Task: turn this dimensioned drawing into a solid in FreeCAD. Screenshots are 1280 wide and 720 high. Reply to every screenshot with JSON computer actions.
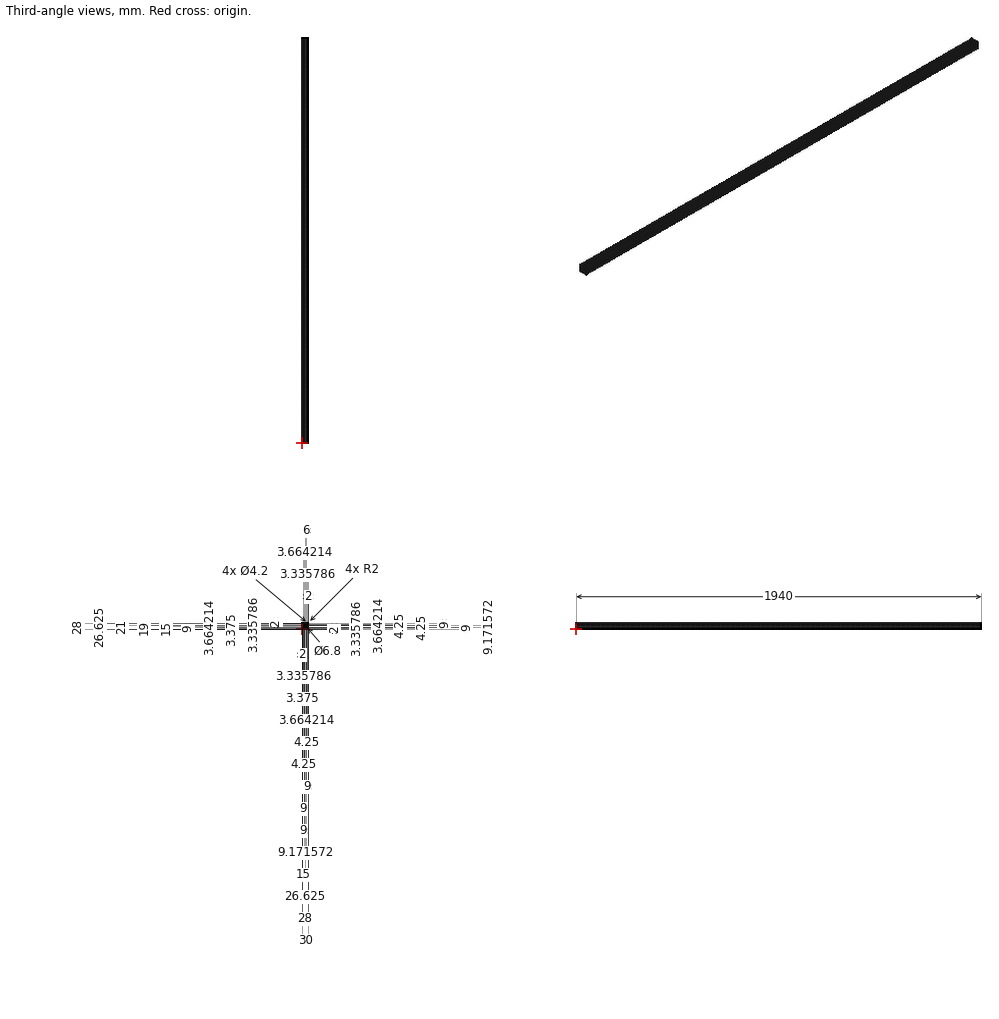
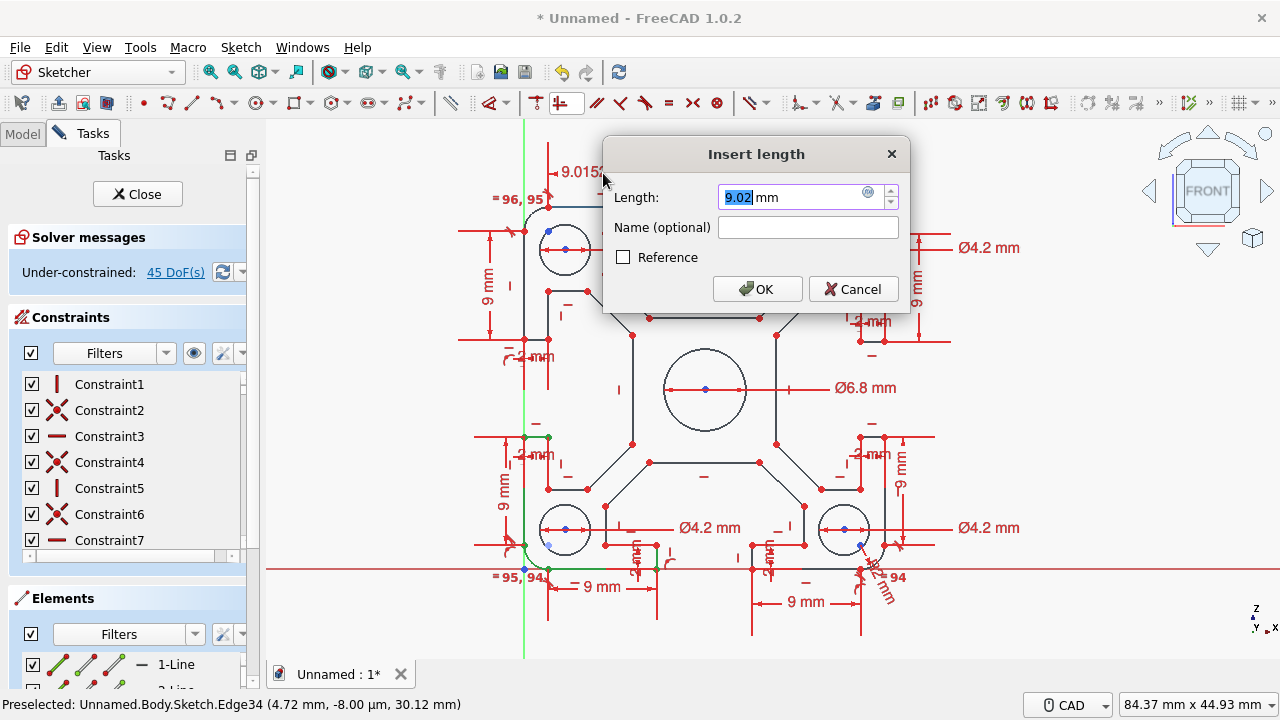
{"action": "type", "text": "9"}
{"action": "key", "text": "Return"}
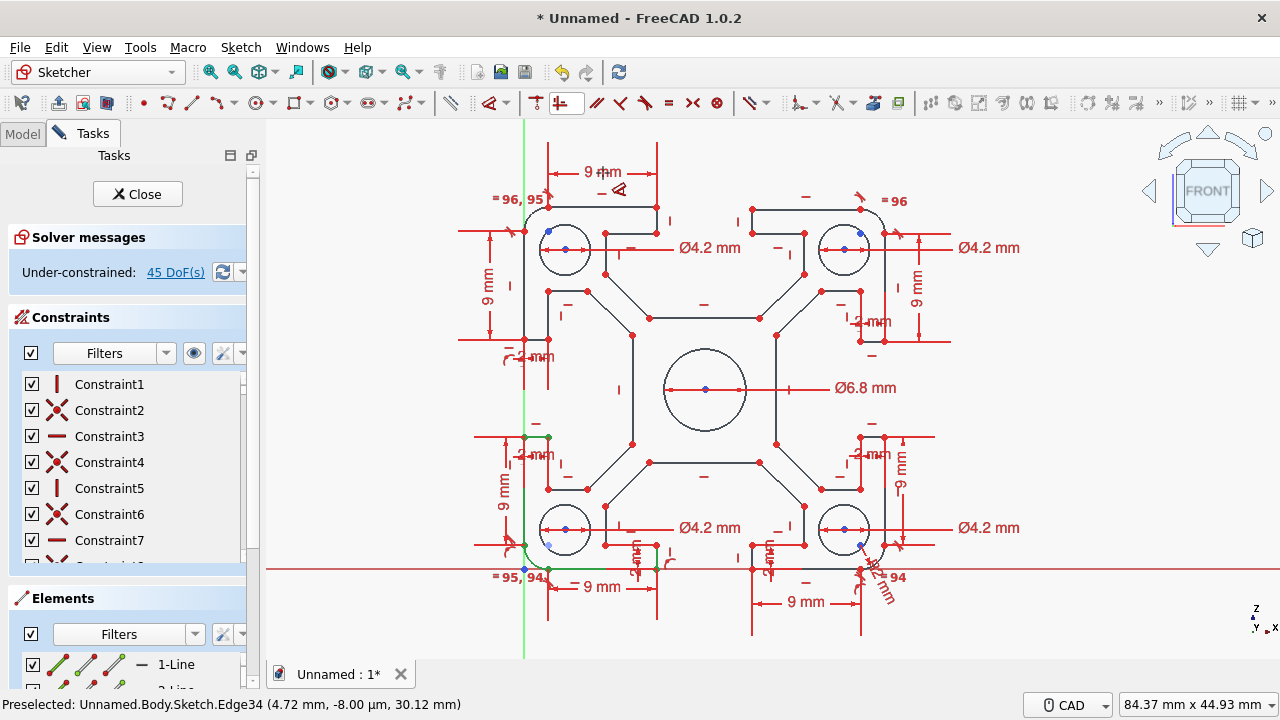
{"action": "scroll", "coordinate": [657, 218], "scroll_direction": "up", "scroll_amount": 3}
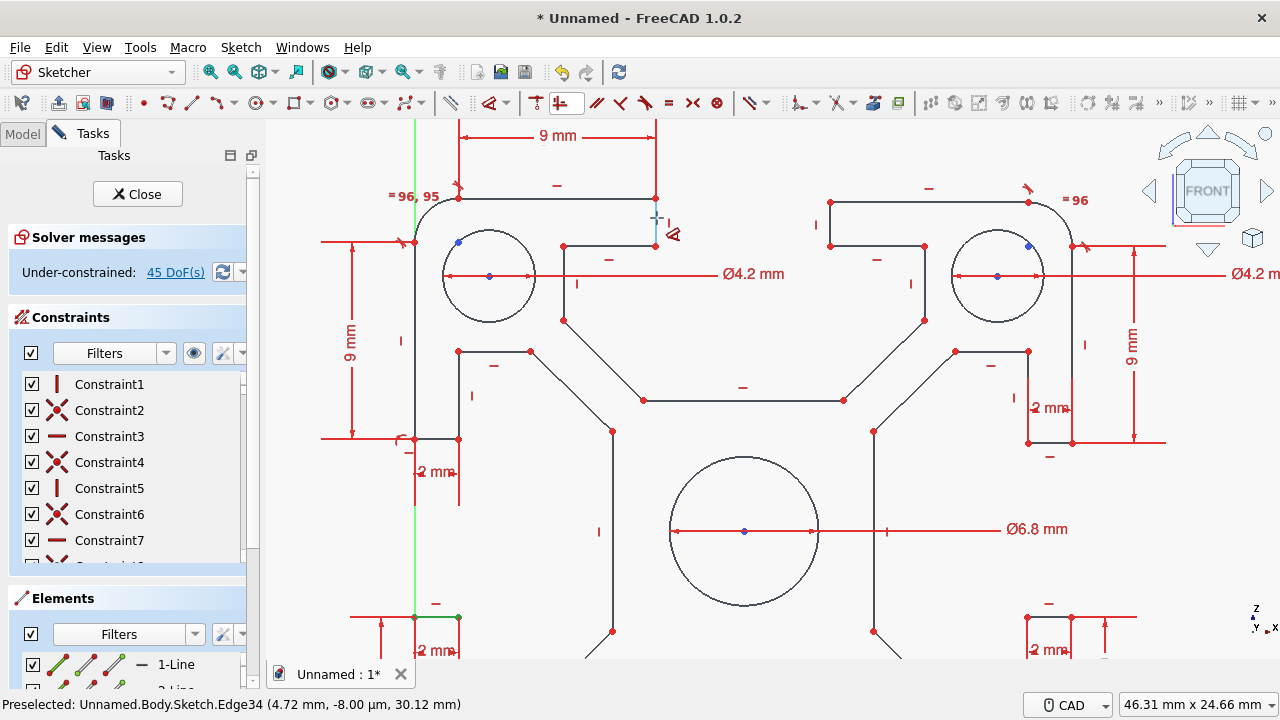
{"action": "left_click", "coordinate": [656, 218]}
{"action": "left_click", "coordinate": [622, 222]}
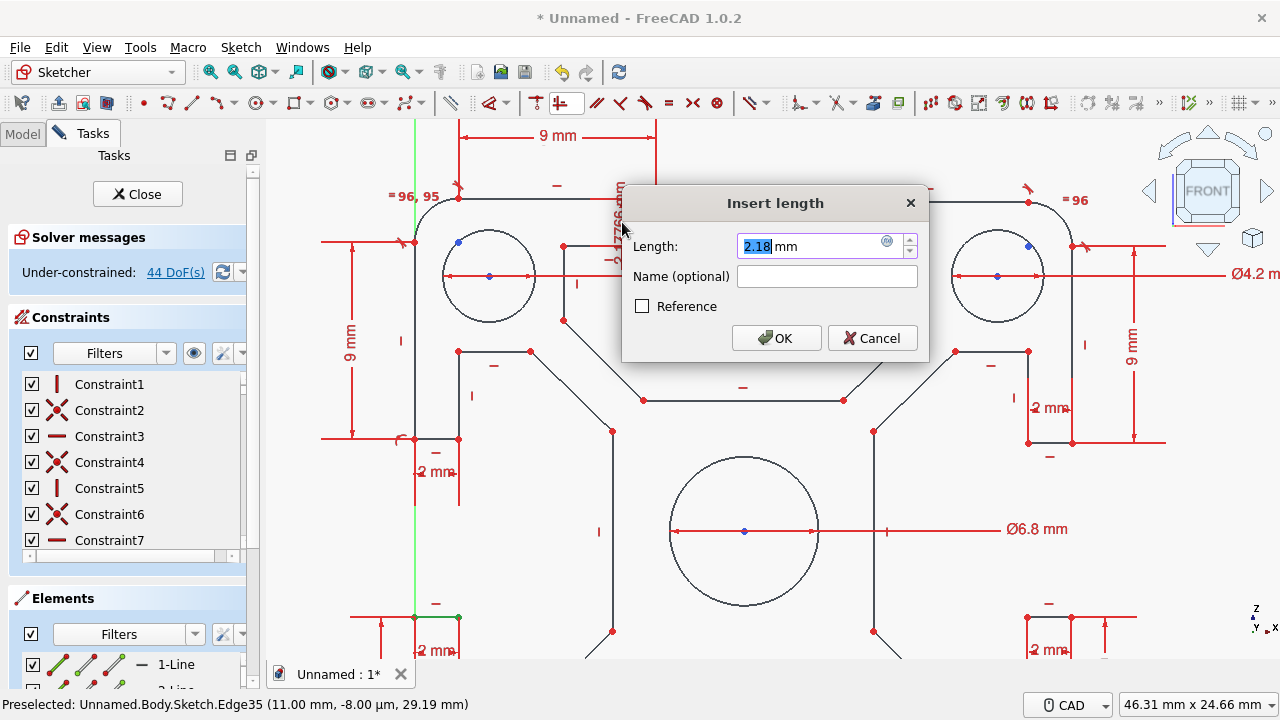
{"action": "type", "text": "2"}
{"action": "key", "text": "Return"}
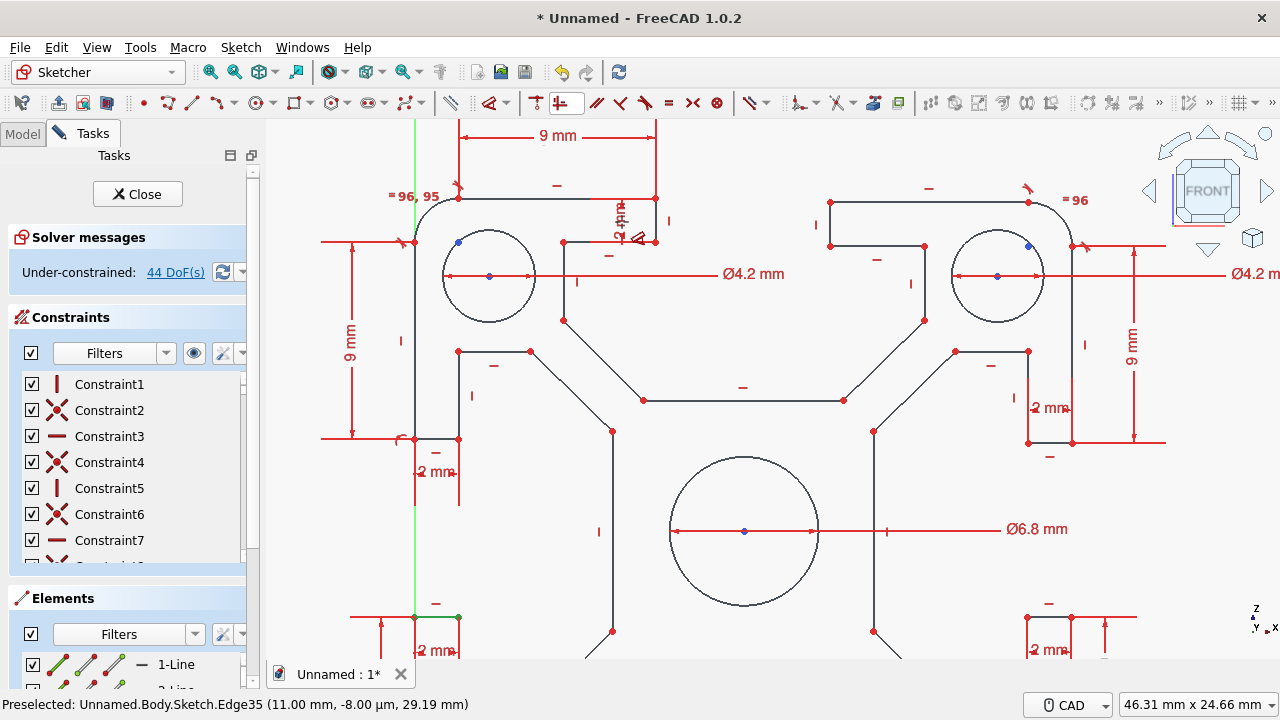
{"action": "left_click", "coordinate": [830, 233]}
{"action": "left_click", "coordinate": [864, 224]}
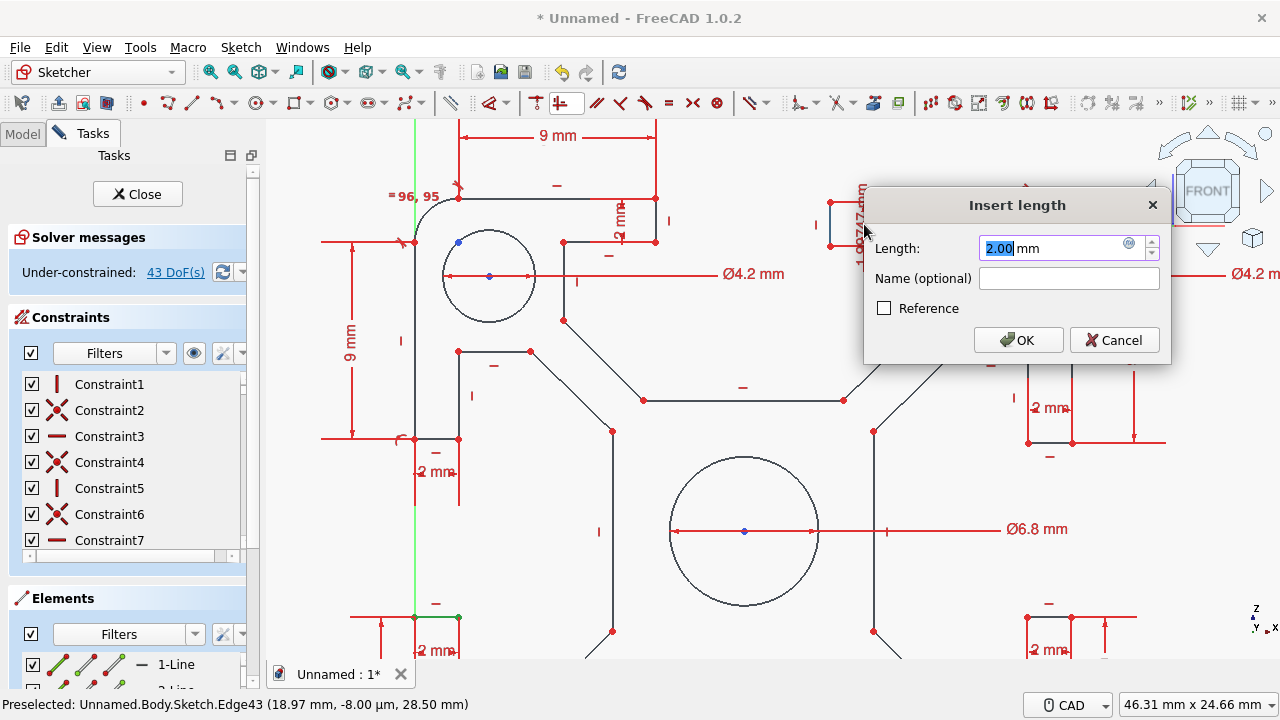
{"action": "type", "text": "2"}
{"action": "key", "text": "Return"}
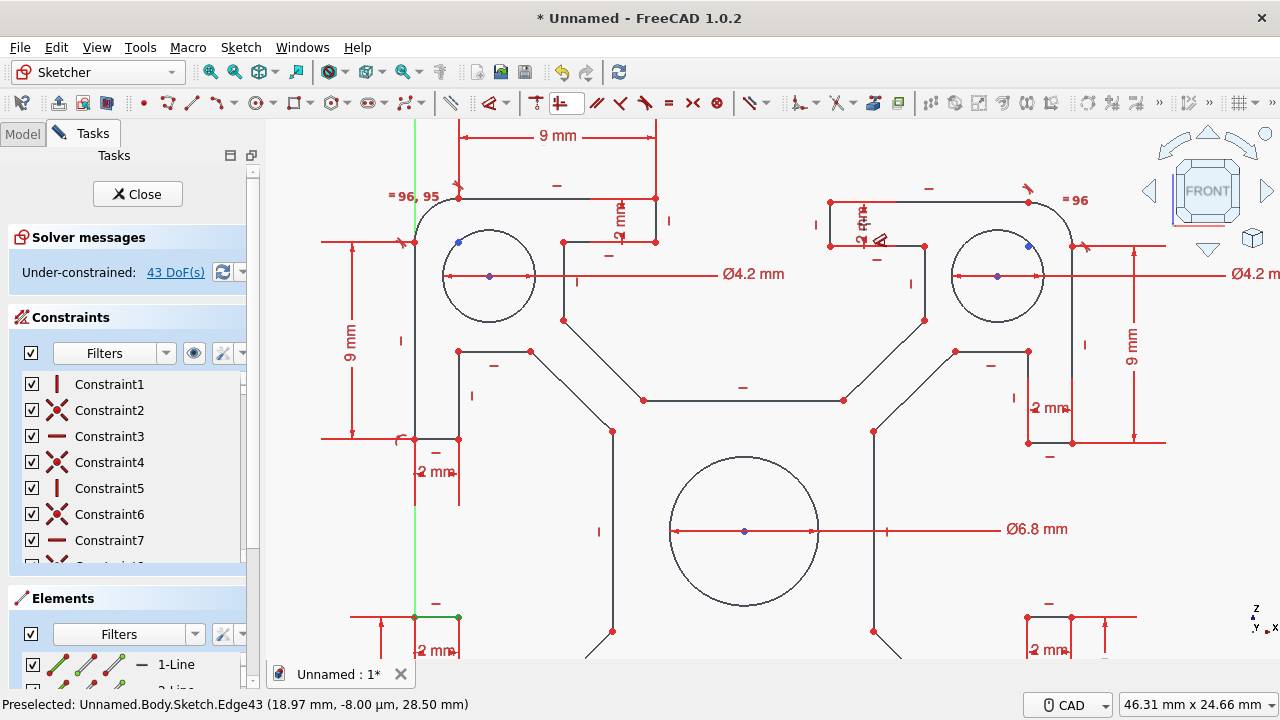
{"action": "left_click", "coordinate": [890, 202]}
{"action": "left_click", "coordinate": [929, 168]}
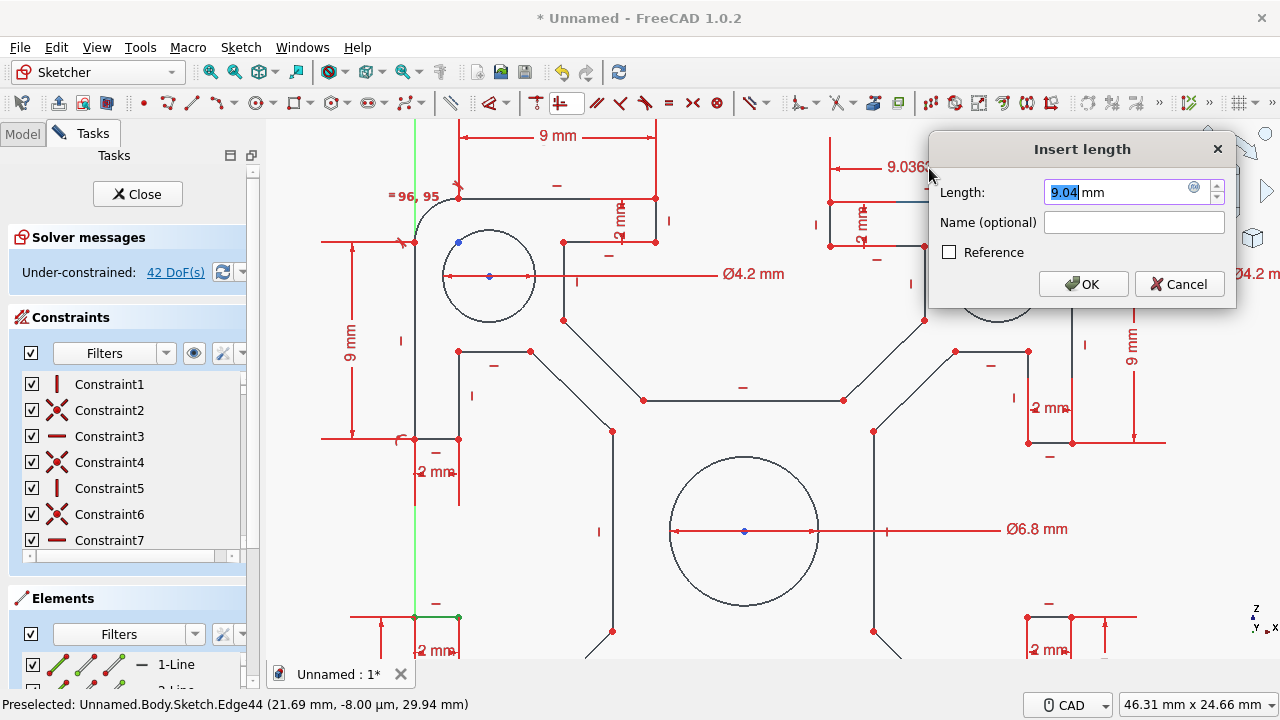
{"action": "type", "text": "9"}
{"action": "key", "text": "Return"}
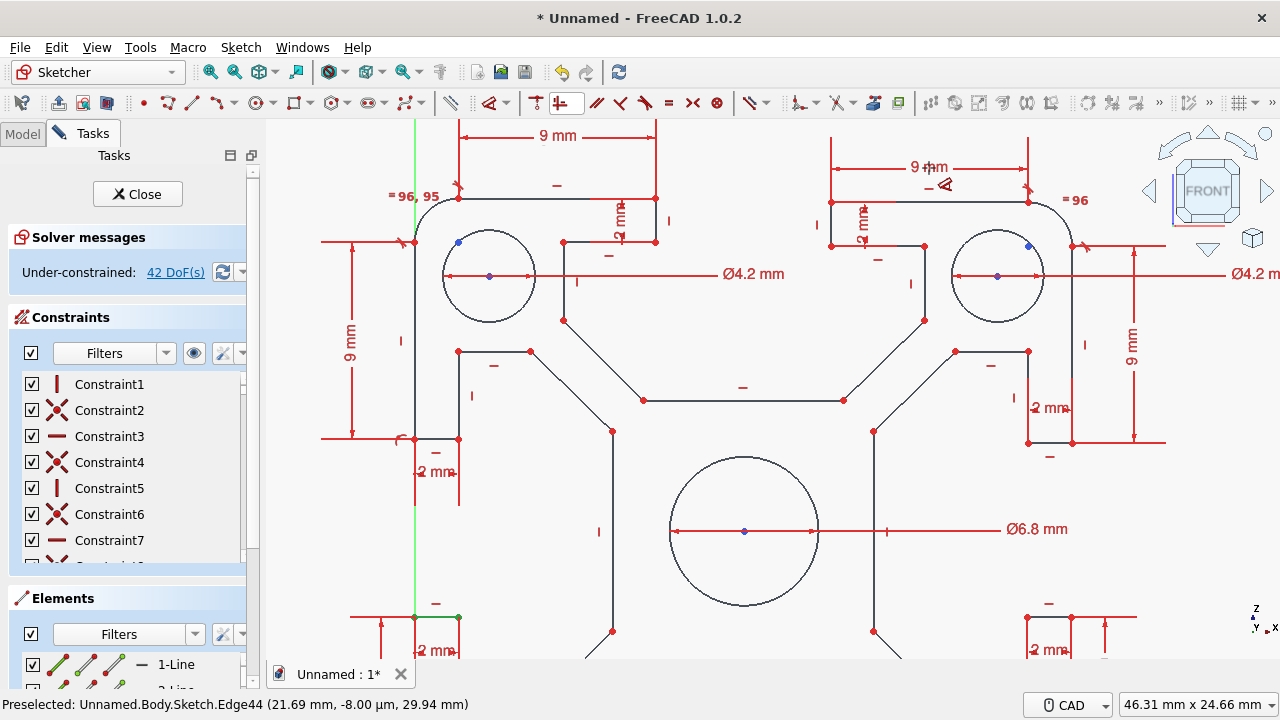
{"action": "scroll", "coordinate": [657, 218], "scroll_direction": "down", "scroll_amount": 3}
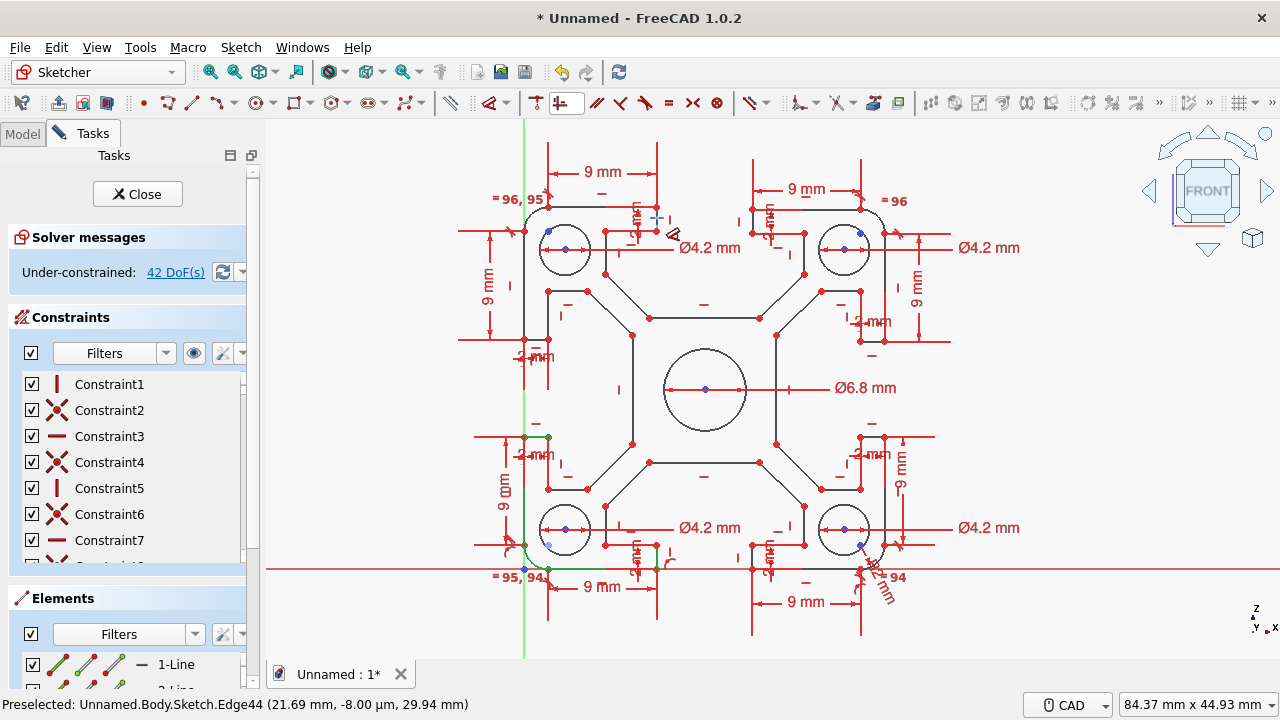
{"action": "left_click", "coordinate": [759, 463]}
{"action": "left_click", "coordinate": [490, 516]}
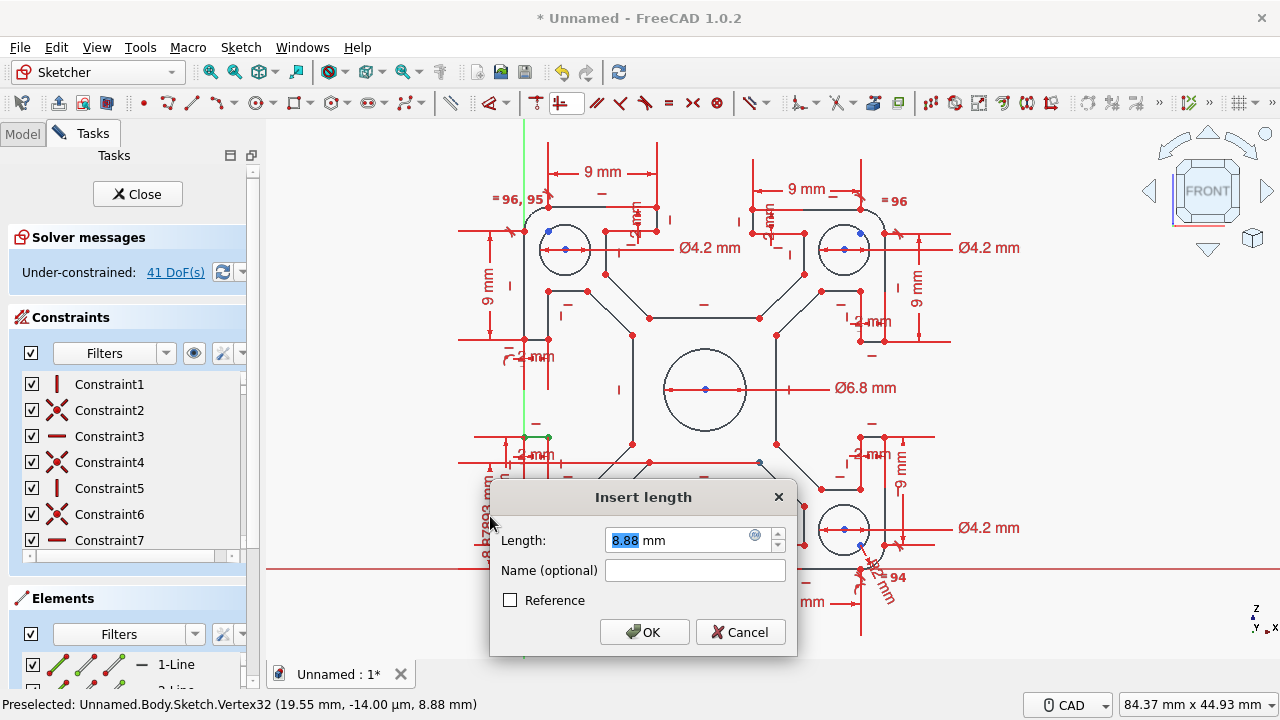
{"action": "type", "text": "9"}
{"action": "key", "text": "Return"}